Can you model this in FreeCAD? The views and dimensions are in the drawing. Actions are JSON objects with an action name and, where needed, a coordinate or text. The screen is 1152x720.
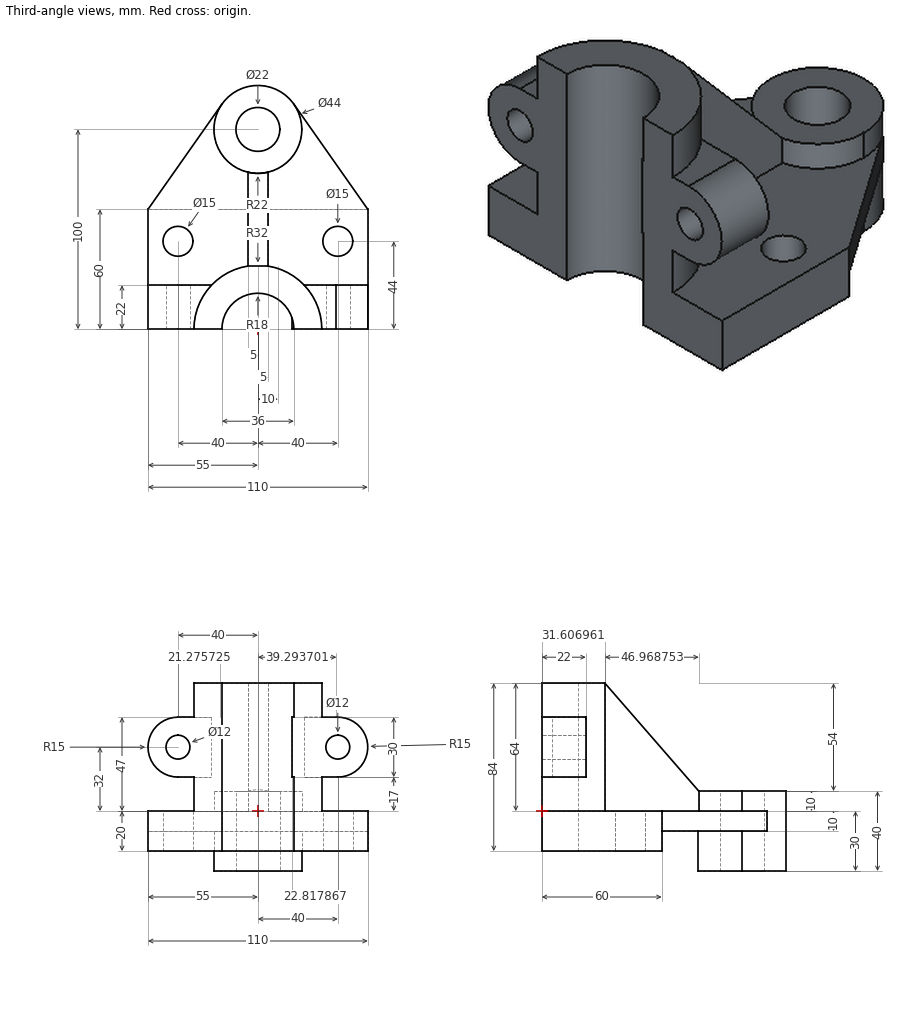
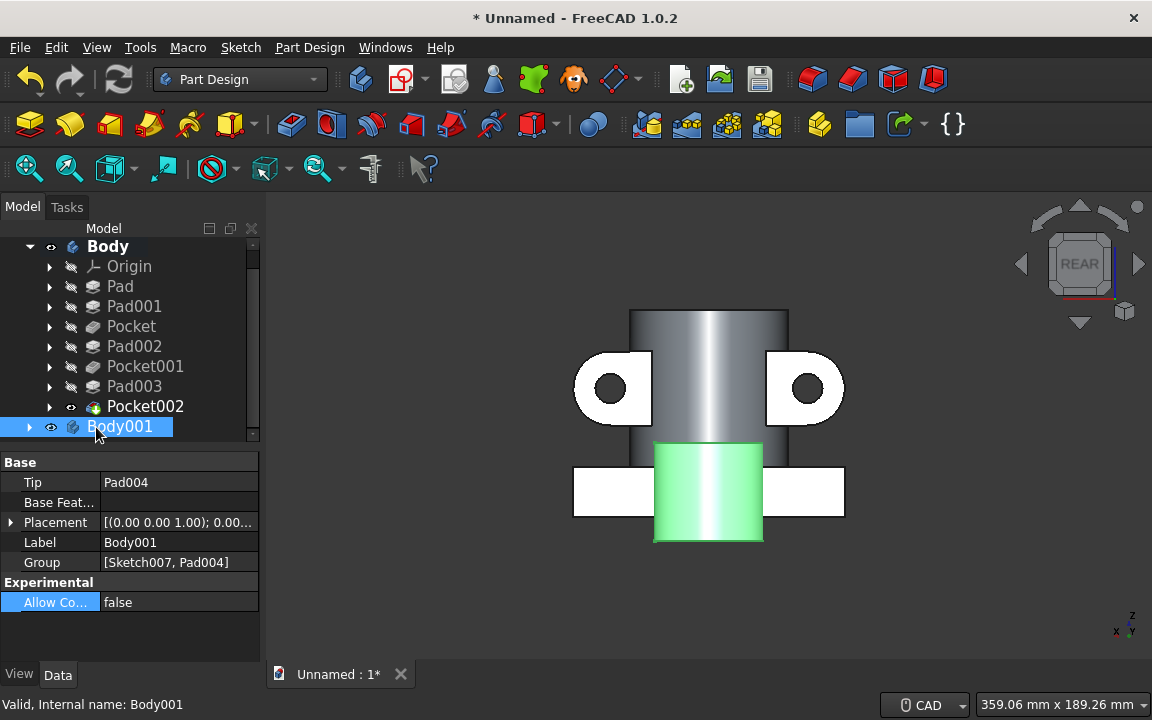
{"action": "left_click", "coordinate": [594, 124]}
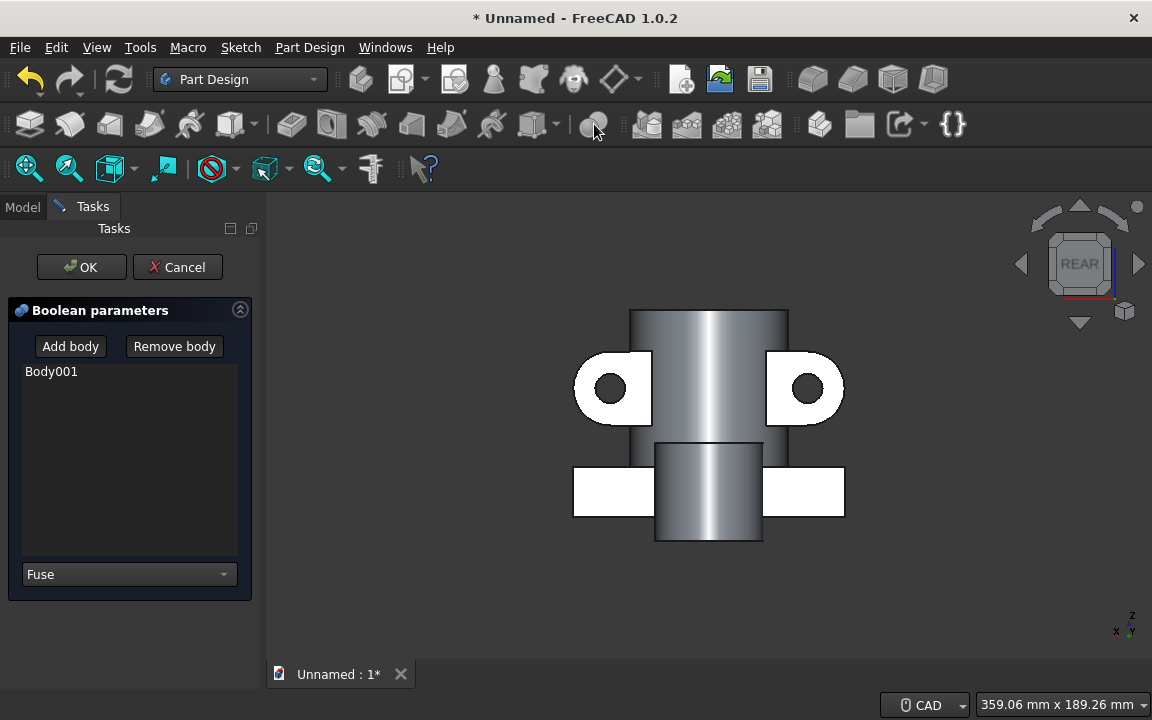
{"action": "left_click", "coordinate": [82, 267]}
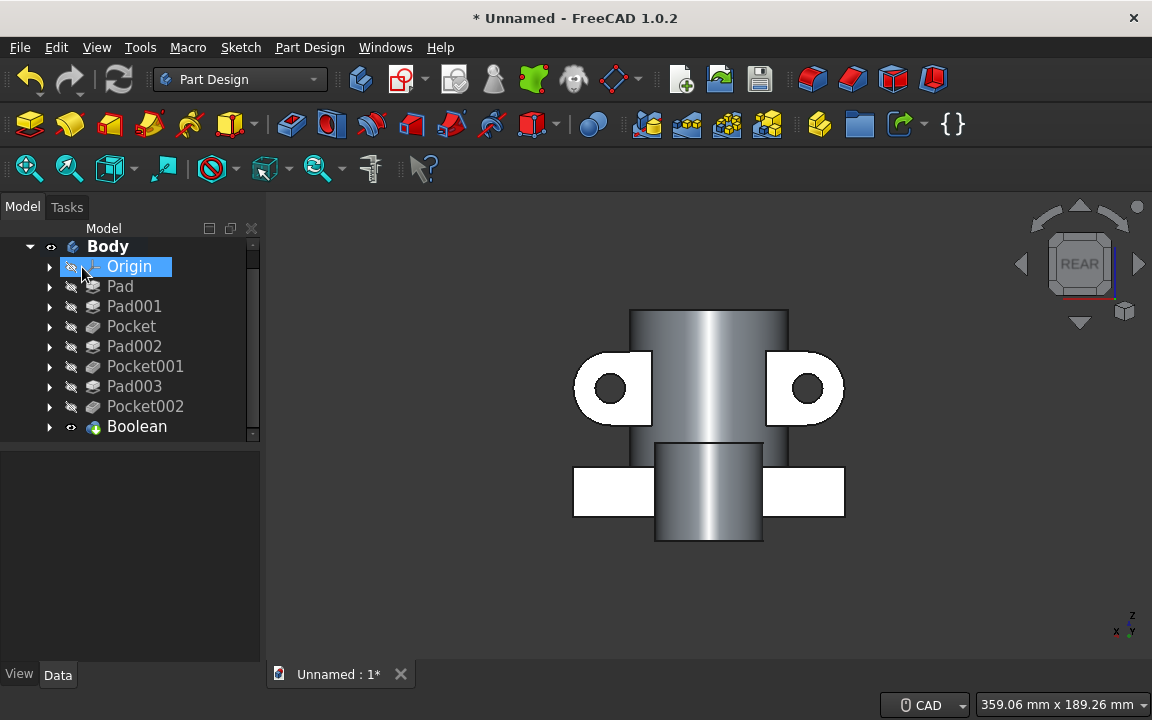
{"action": "left_click", "coordinate": [402, 80]}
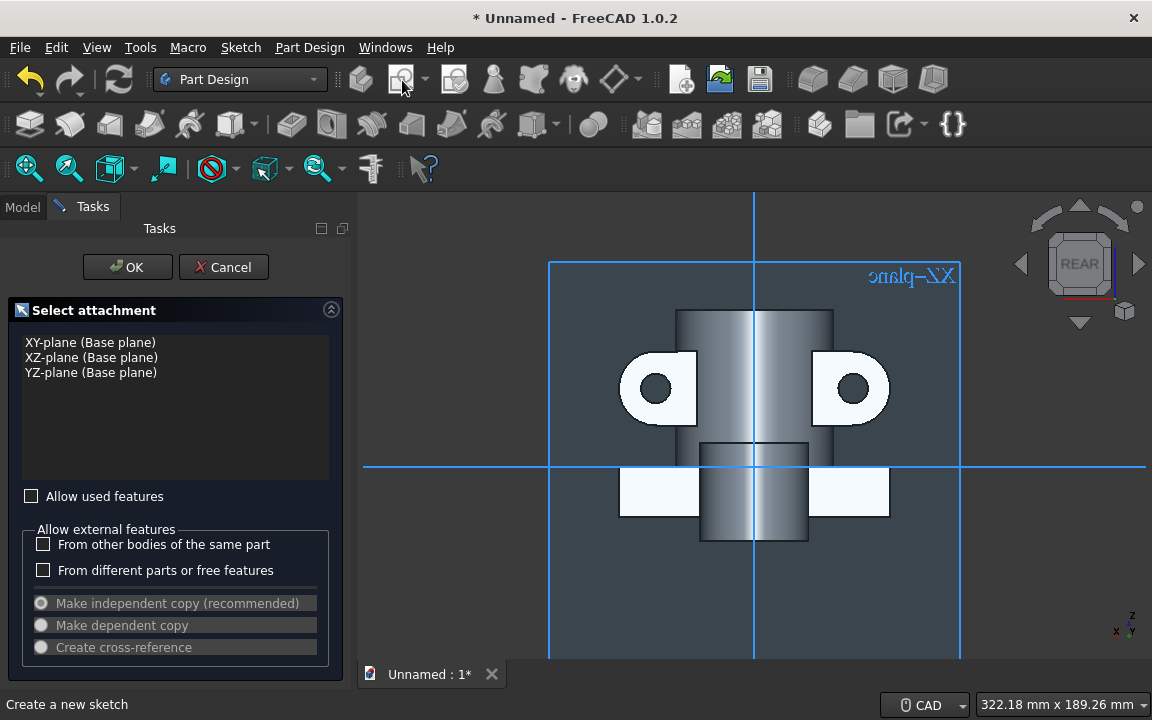
{"action": "left_click", "coordinate": [82, 342]}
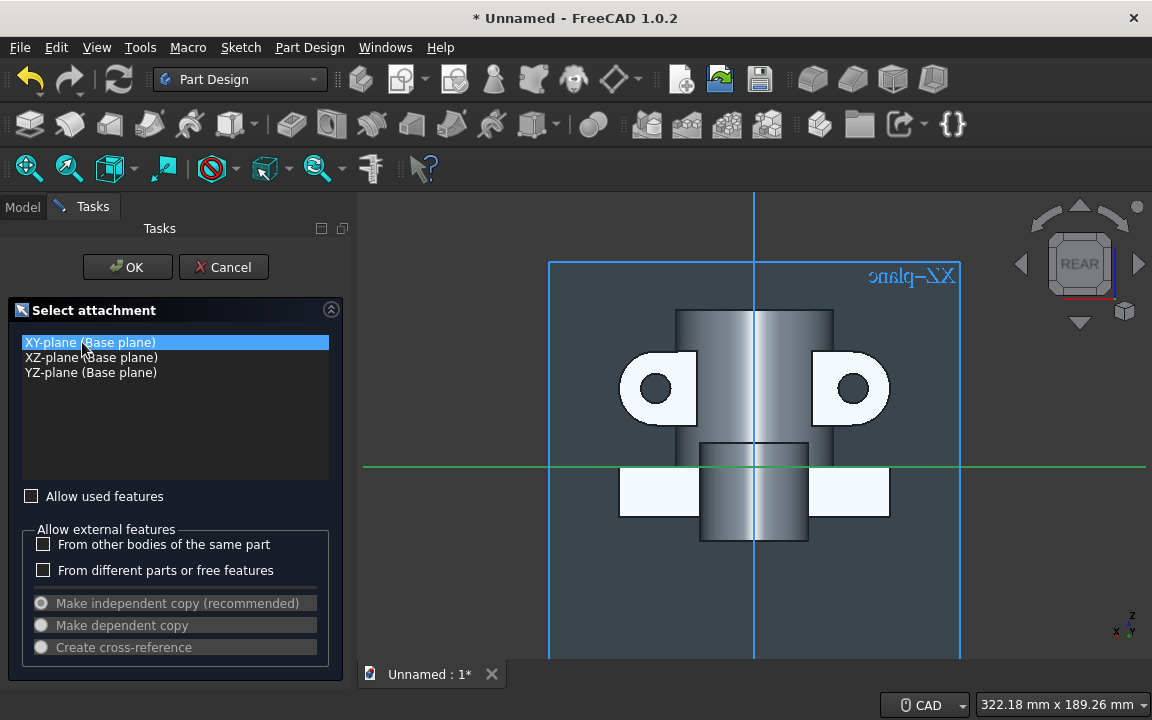
{"action": "left_click", "coordinate": [128, 267]}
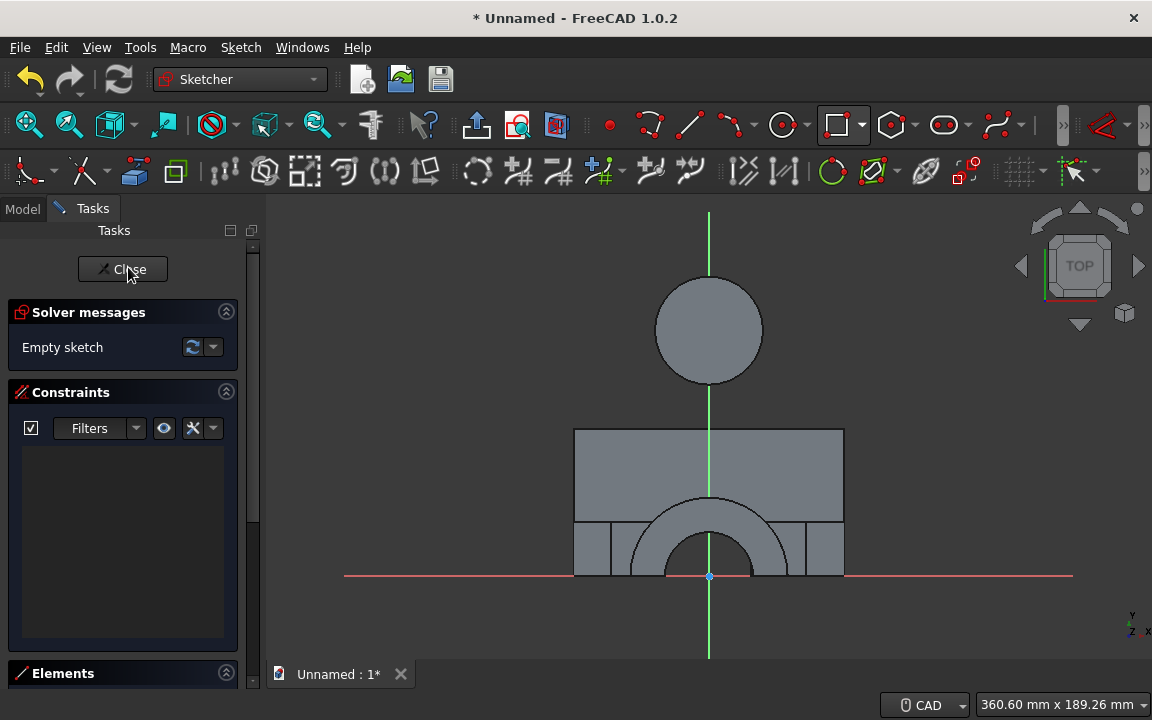
{"action": "left_click", "coordinate": [558, 126]}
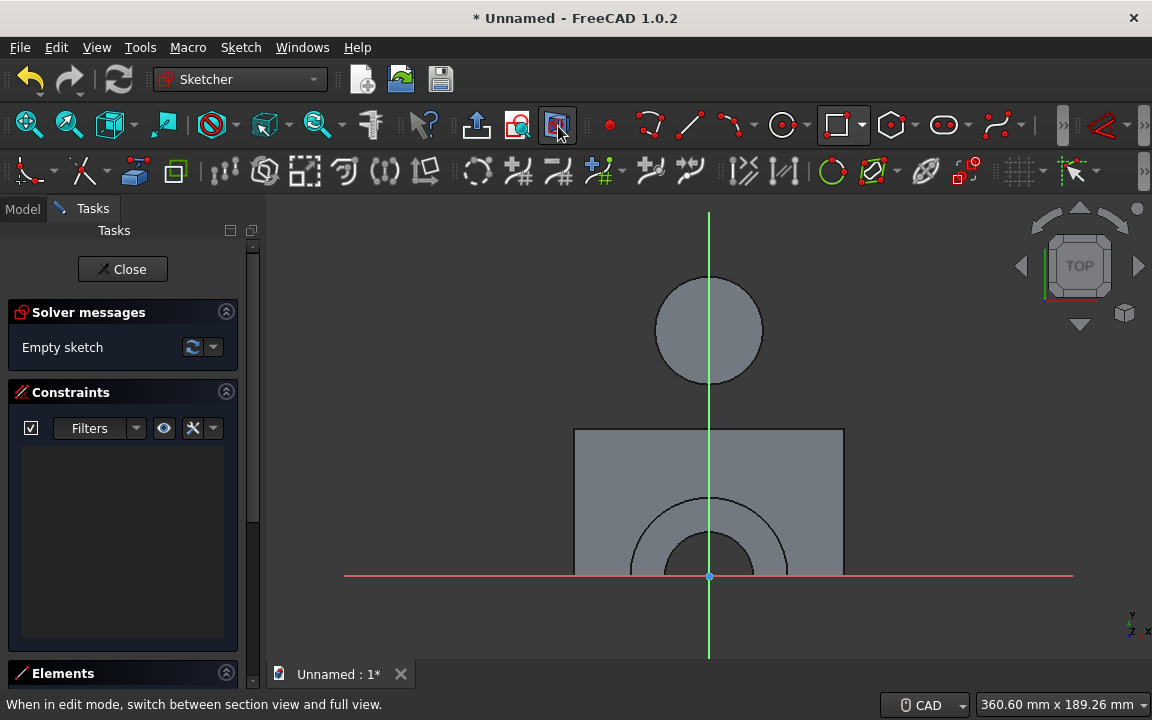
{"action": "left_click", "coordinate": [650, 126]}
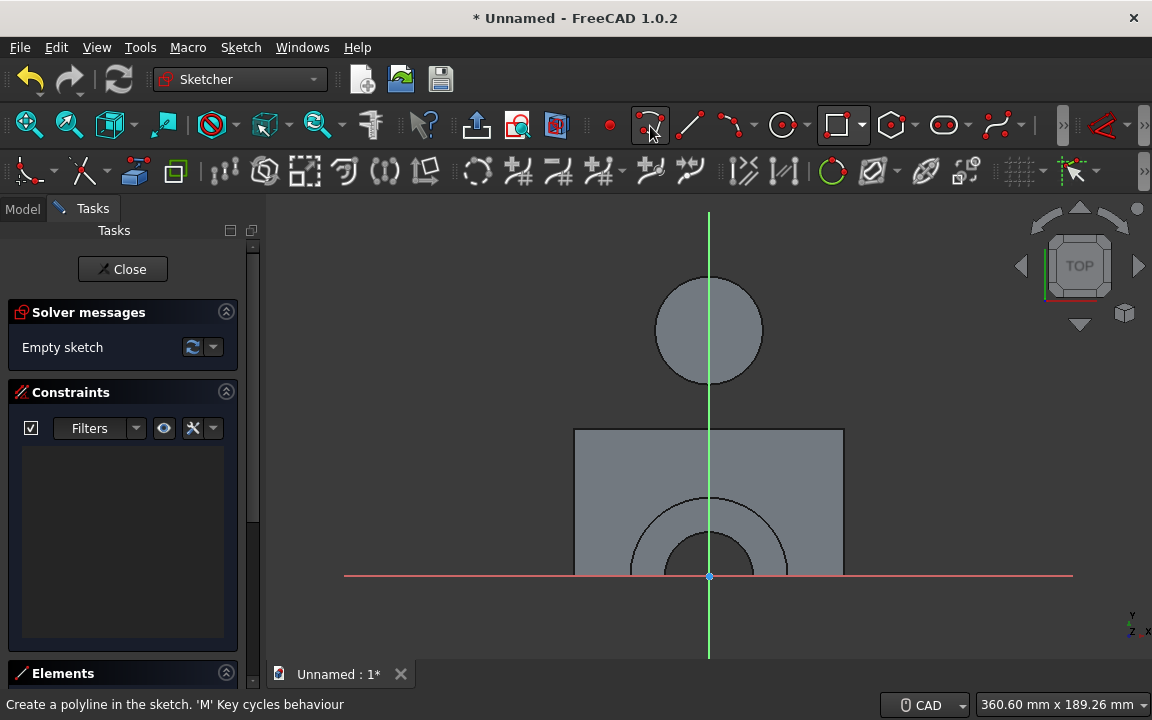
{"action": "left_click", "coordinate": [665, 300]}
{"action": "left_click", "coordinate": [574, 429]}
{"action": "left_click", "coordinate": [844, 429]}
{"action": "left_click", "coordinate": [753, 300]}
{"action": "right_click", "coordinate": [753, 300]}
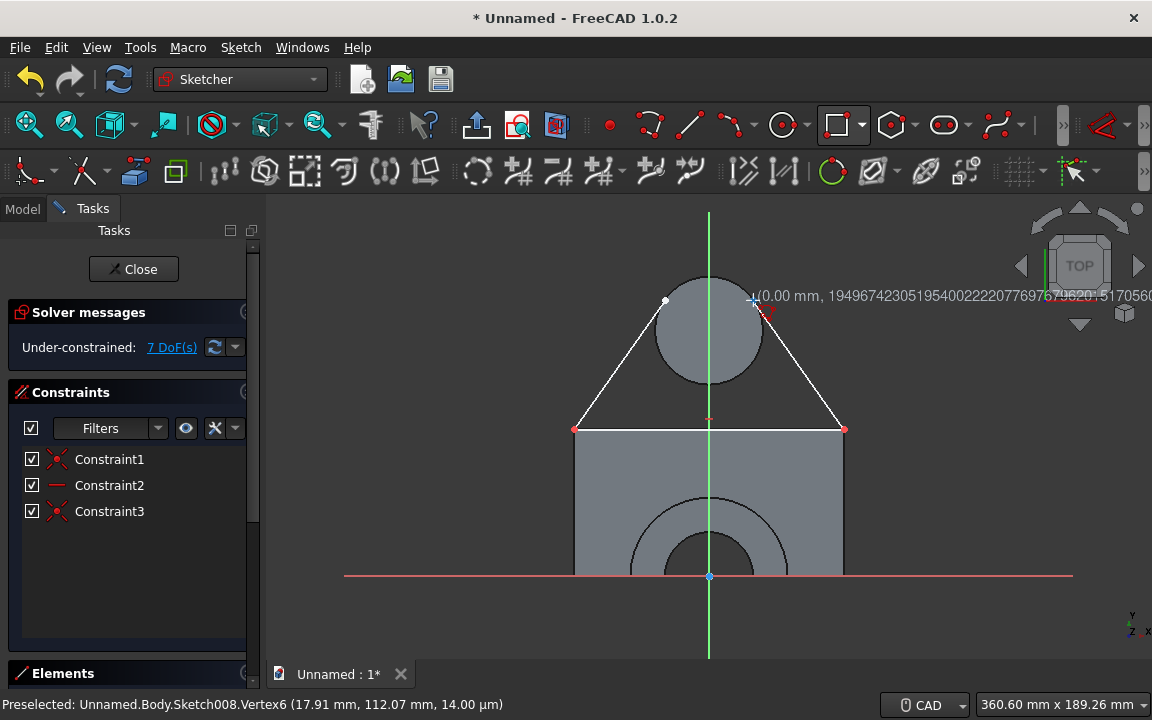
{"action": "left_click", "coordinate": [730, 126]}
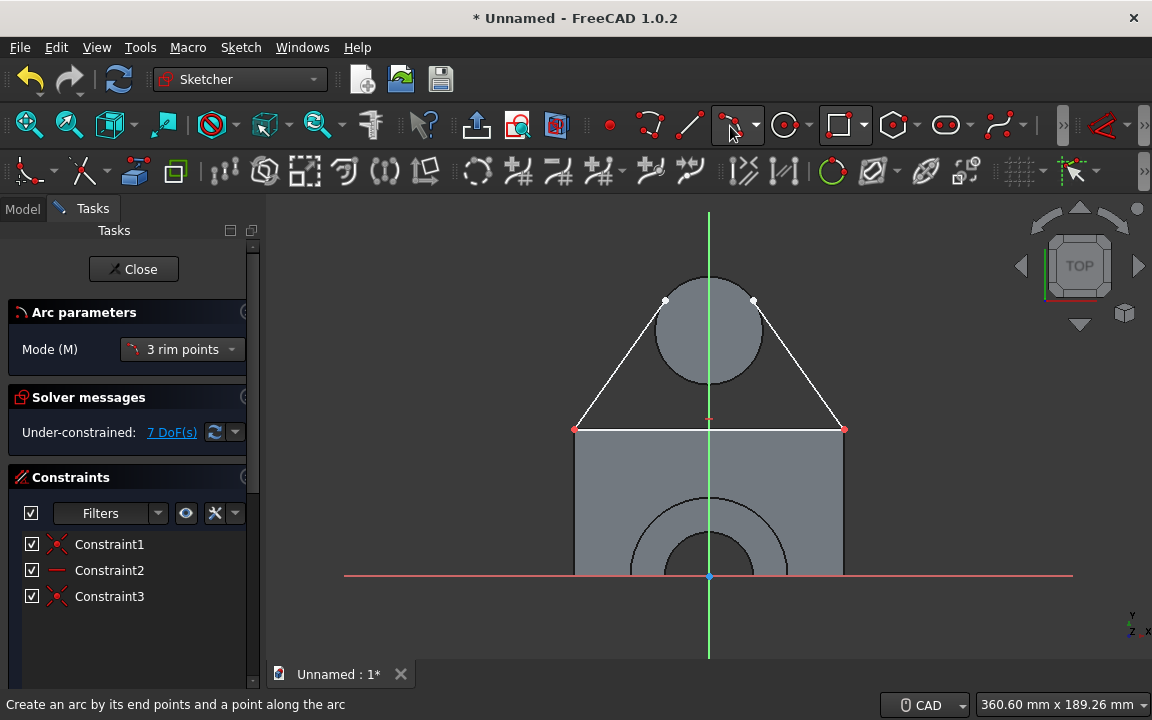
{"action": "left_click", "coordinate": [753, 301]}
{"action": "left_click", "coordinate": [665, 301]}
{"action": "left_click", "coordinate": [686, 380]}
{"action": "key", "text": "Escape"}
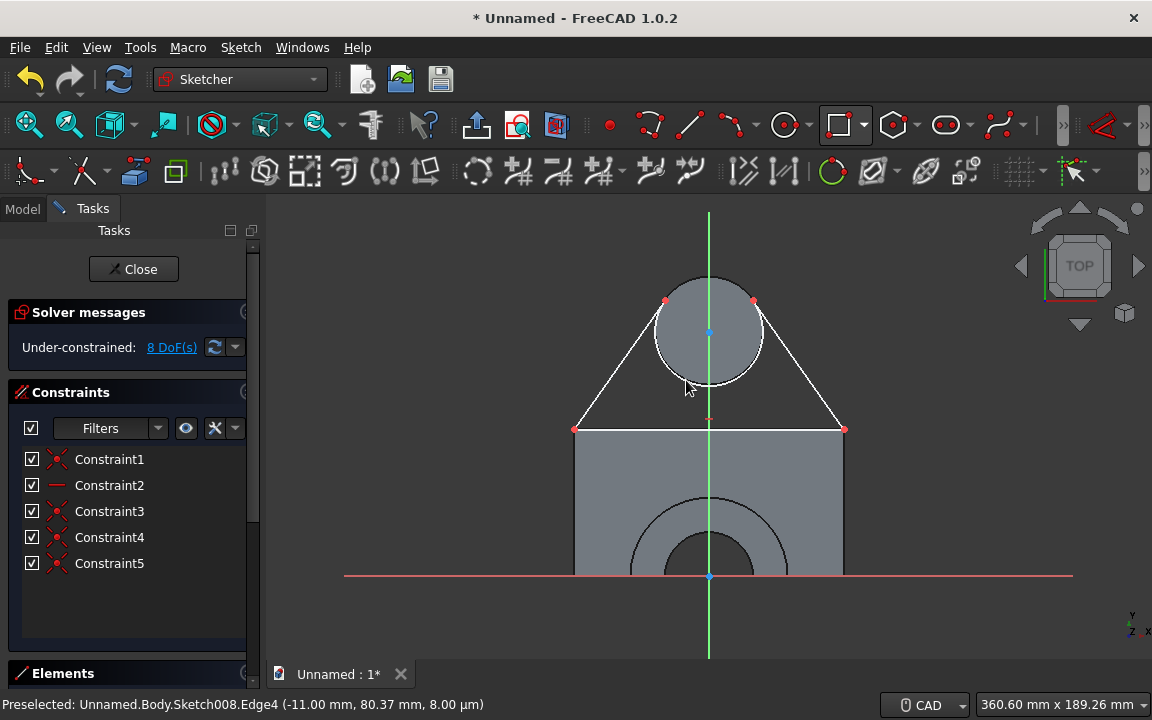
{"action": "left_click", "coordinate": [638, 340]}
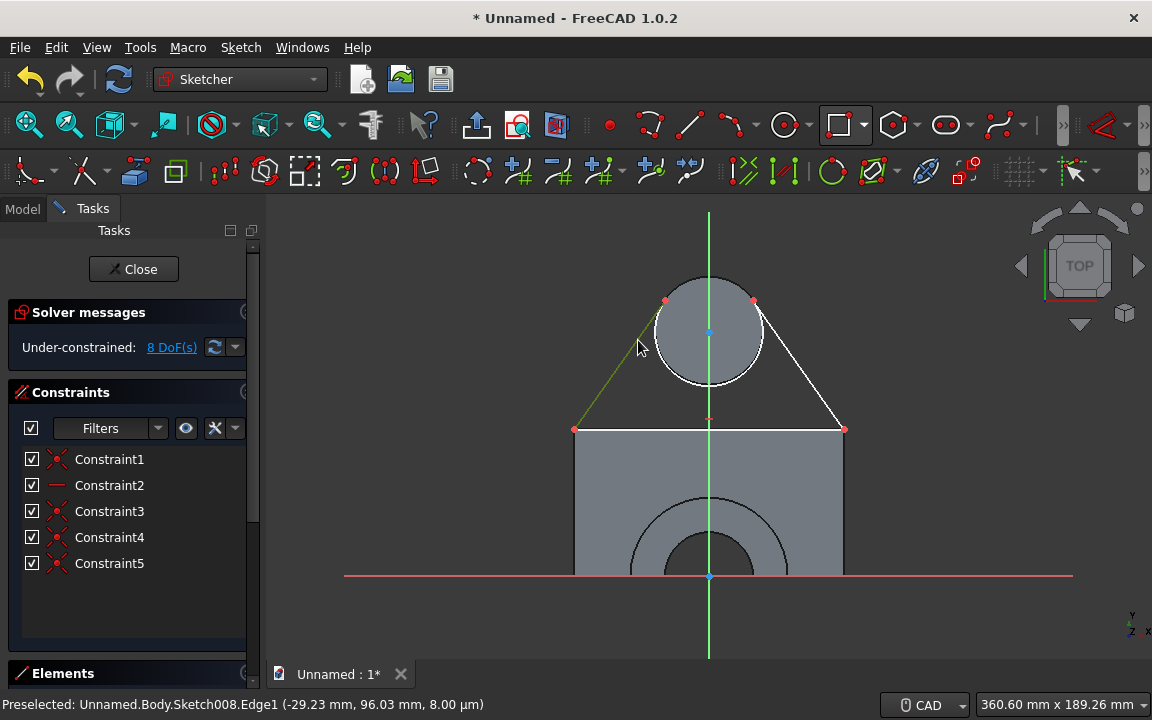
{"action": "left_click", "coordinate": [668, 367]}